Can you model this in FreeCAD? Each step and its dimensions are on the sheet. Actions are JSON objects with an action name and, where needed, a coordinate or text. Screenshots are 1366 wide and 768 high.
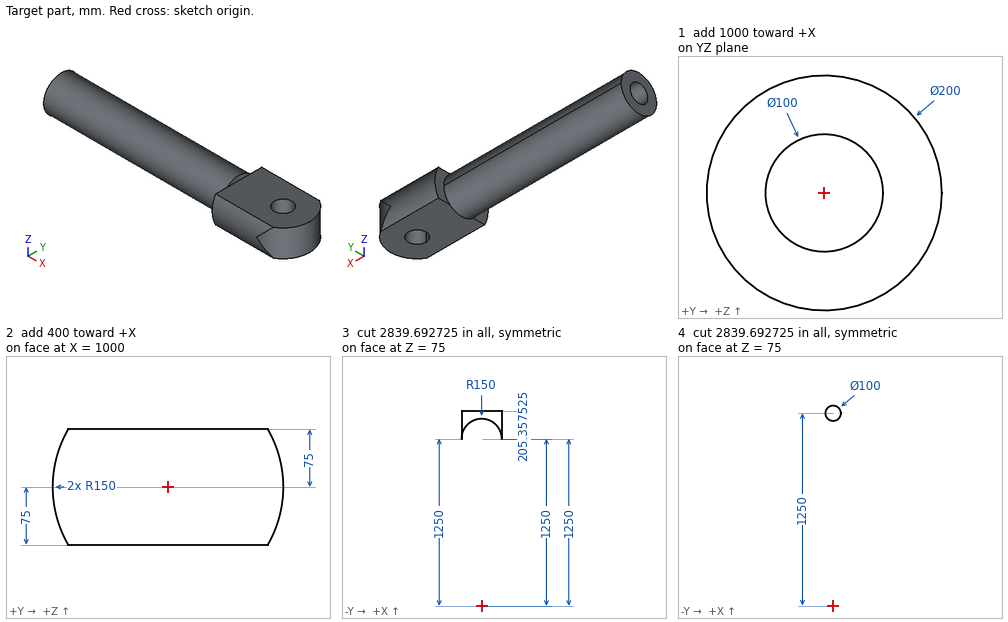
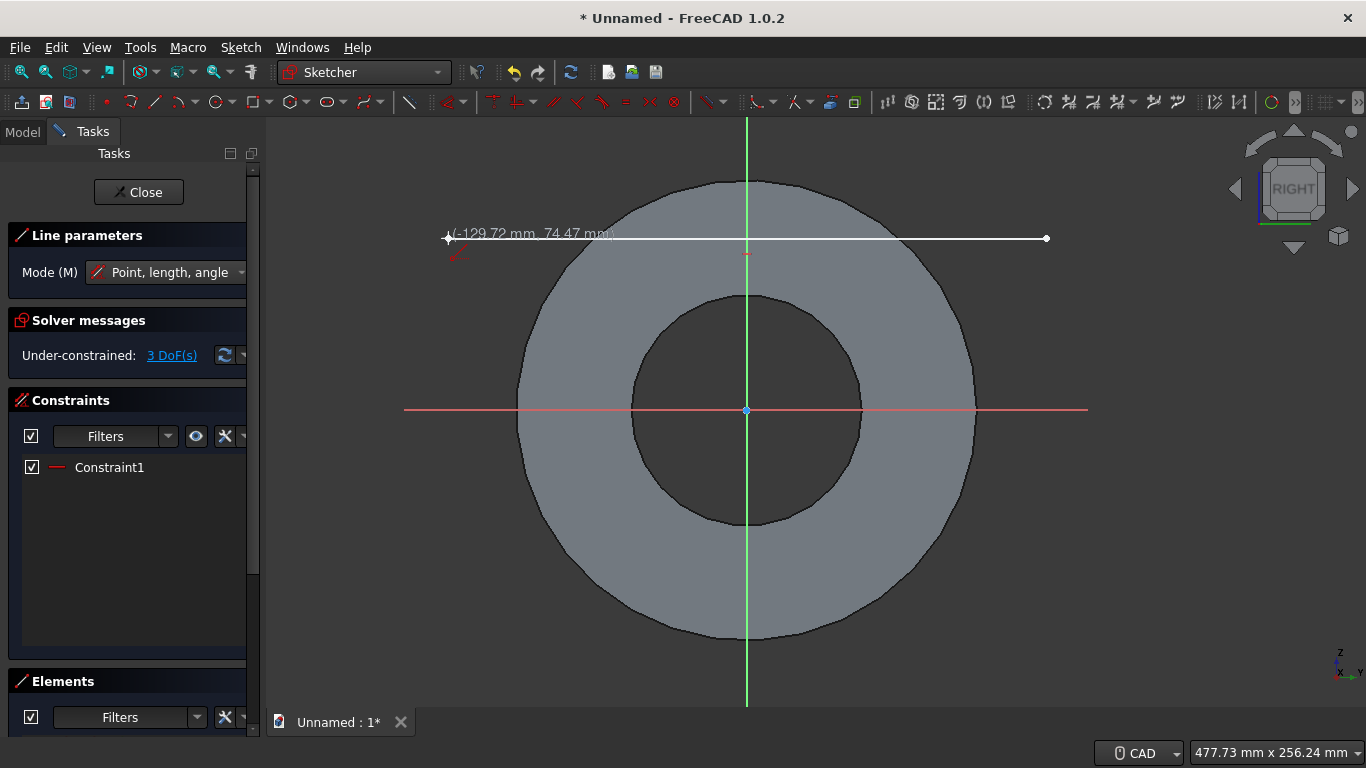
{"action": "left_click", "coordinate": [448, 583]}
{"action": "left_click", "coordinate": [1046, 583]}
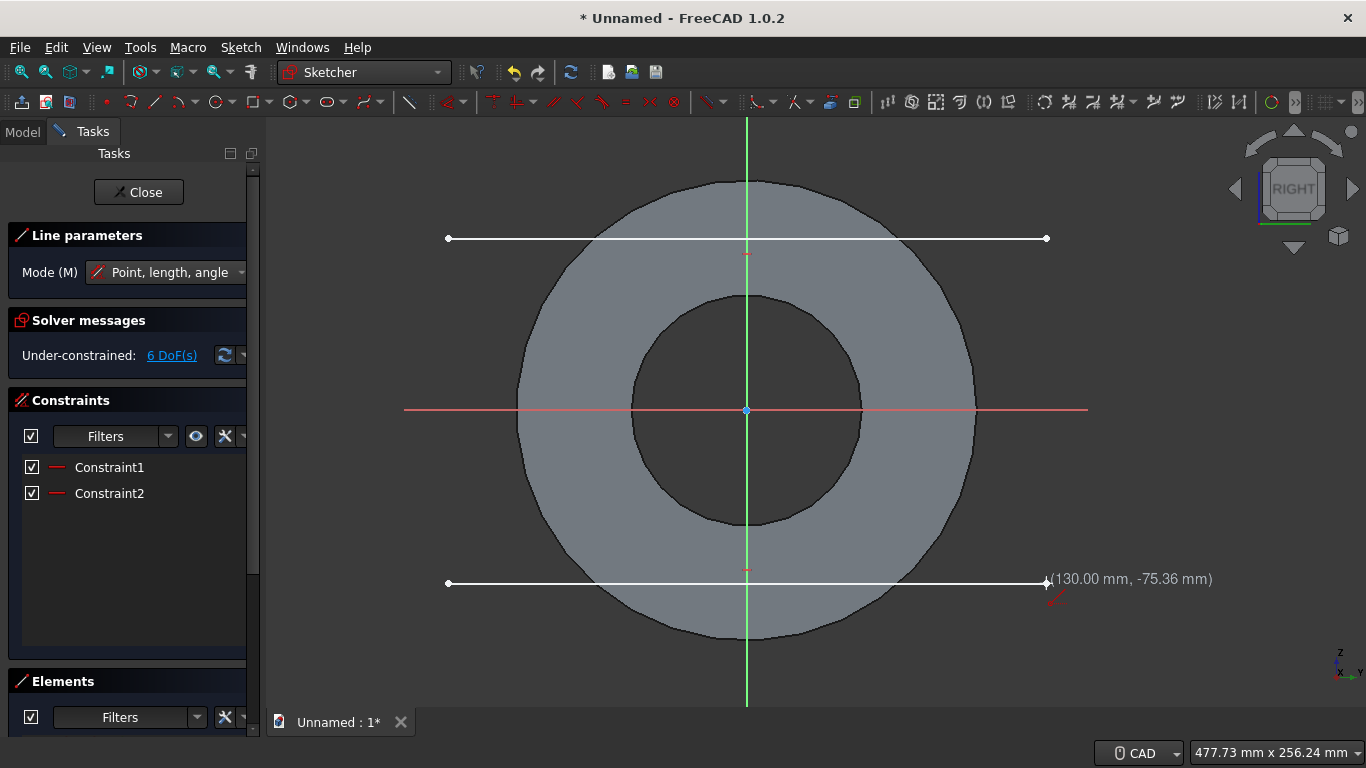
{"action": "key", "text": "g 3 a"}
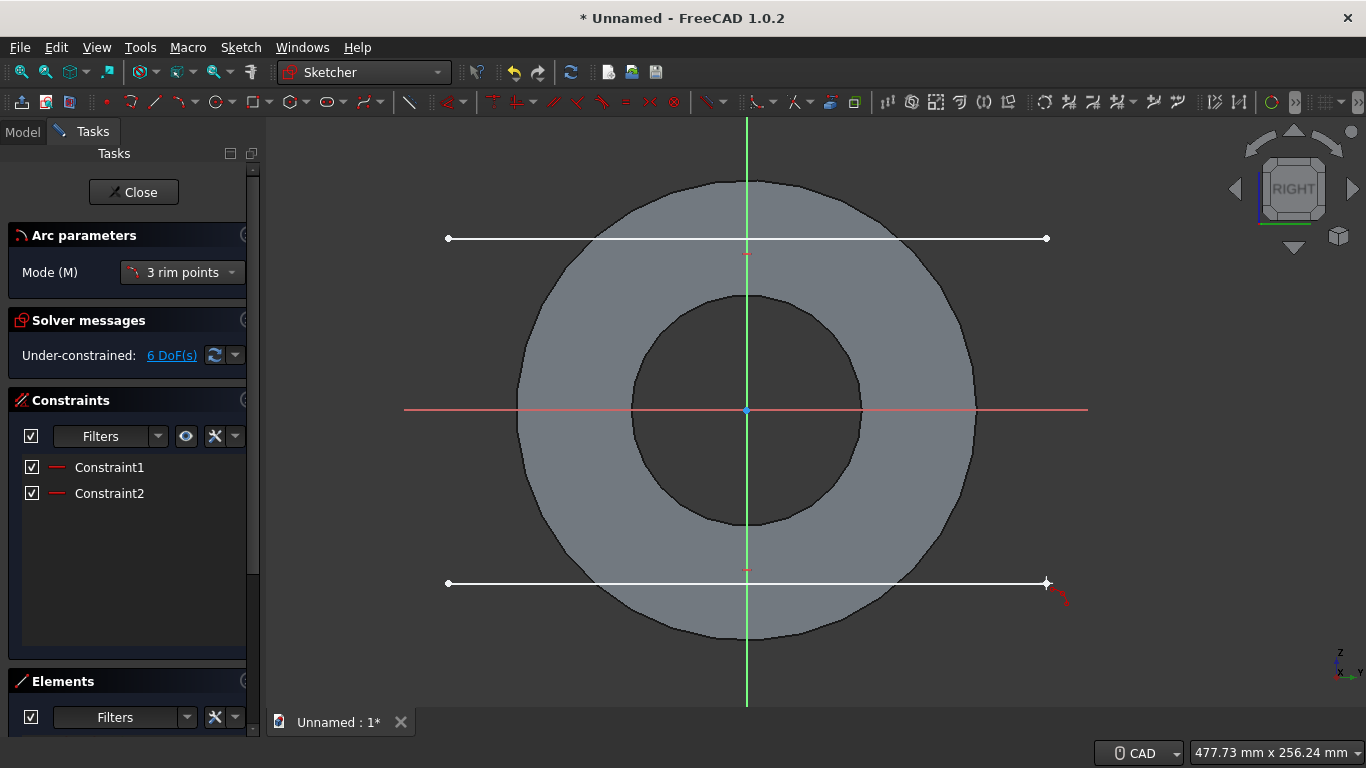
{"action": "left_click", "coordinate": [448, 239]}
{"action": "left_click", "coordinate": [448, 584]}
{"action": "left_click", "coordinate": [403, 374]}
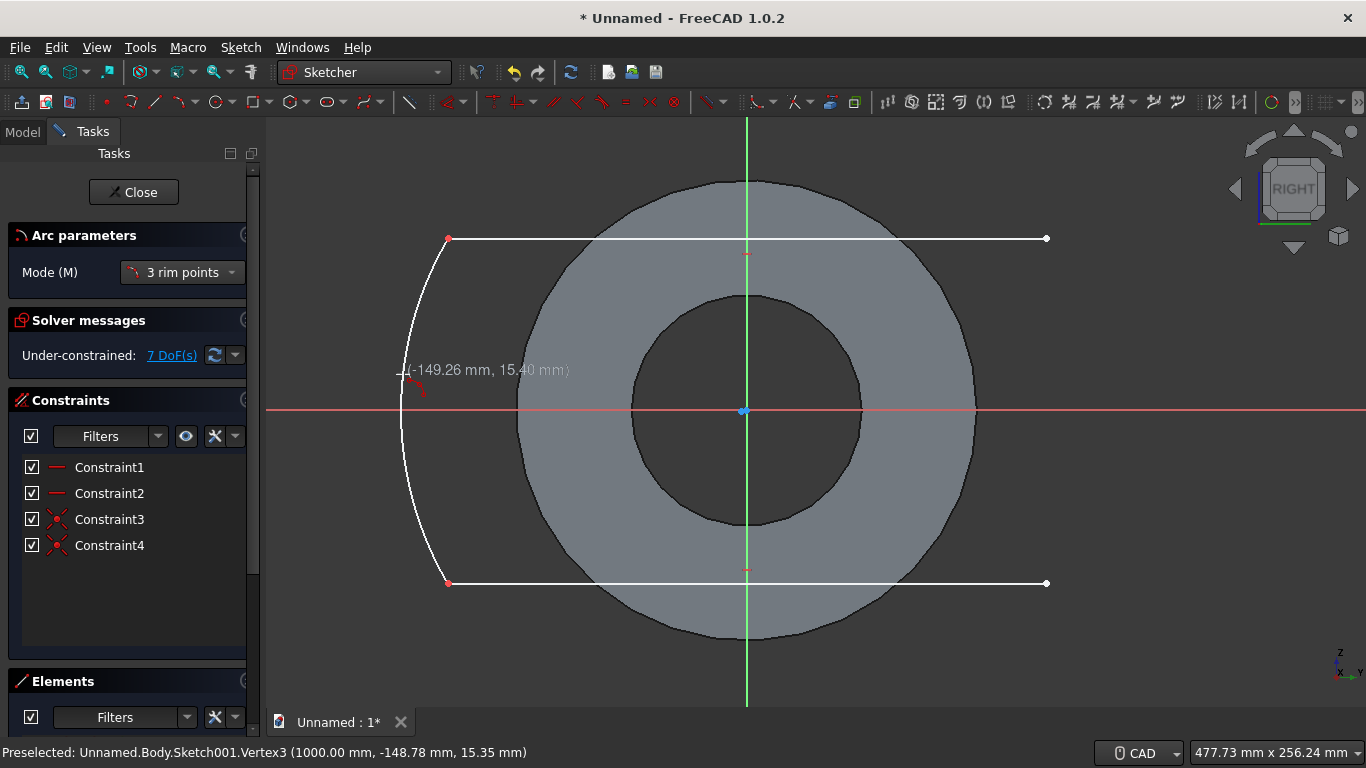
{"action": "left_click", "coordinate": [1046, 584]}
{"action": "left_click", "coordinate": [1046, 239]}
{"action": "left_click", "coordinate": [1090, 447]}
{"action": "key", "text": "Escape"}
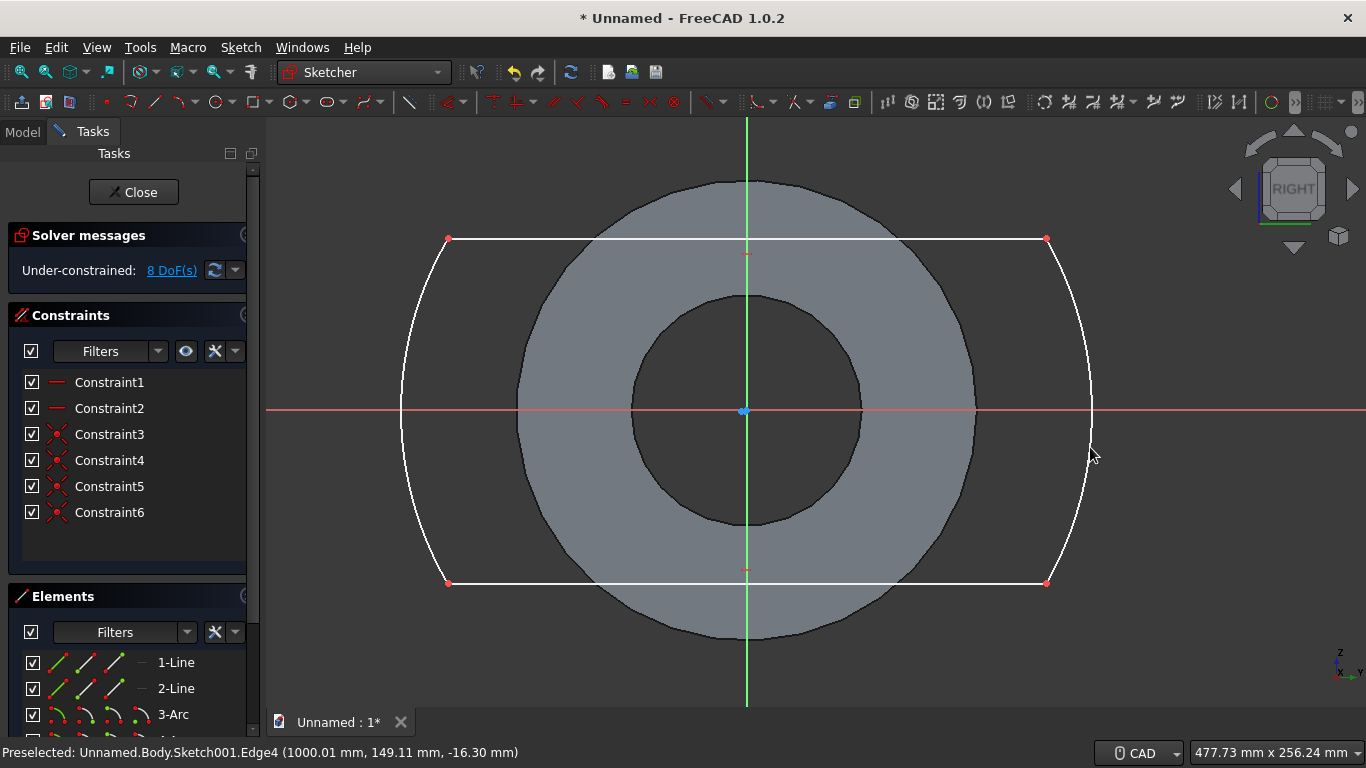
{"action": "left_click", "coordinate": [409, 340]}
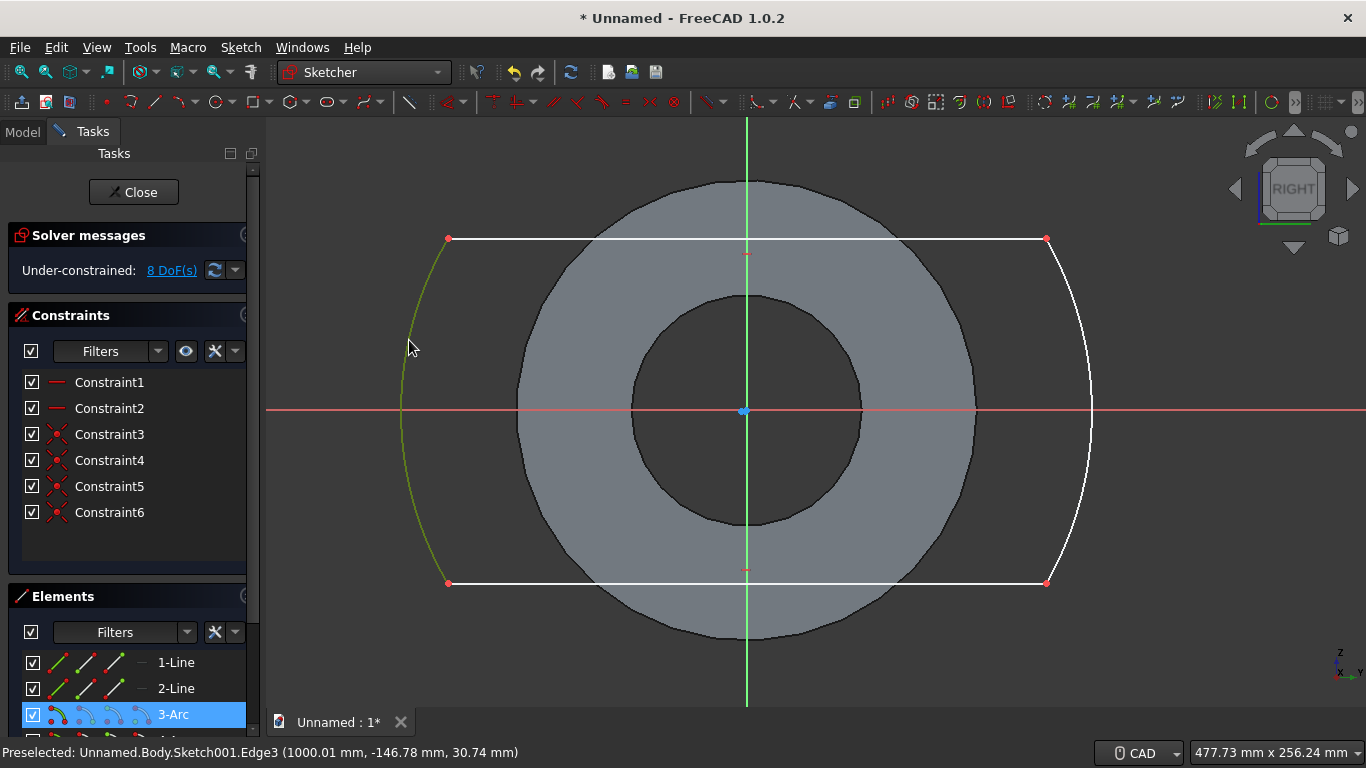
{"action": "left_click", "coordinate": [1084, 483]}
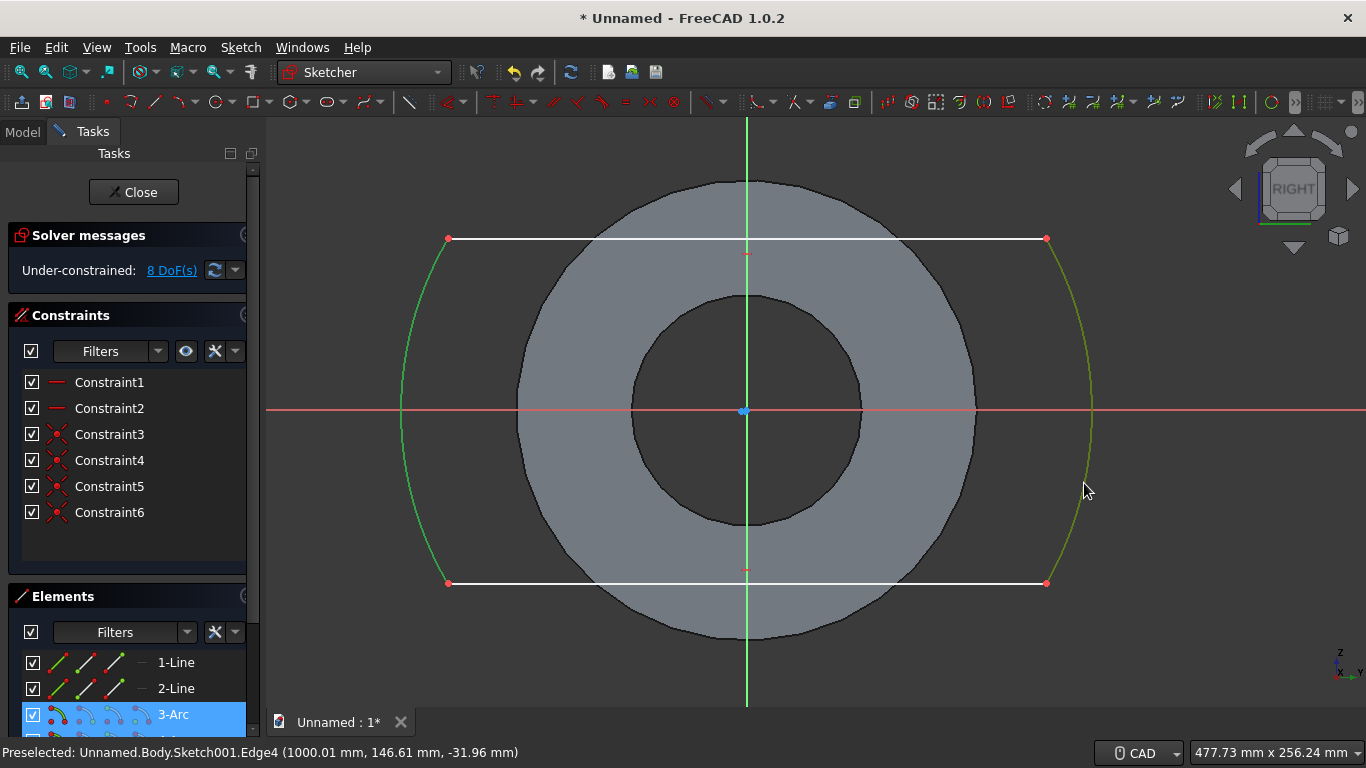
{"action": "left_click", "coordinate": [494, 102]}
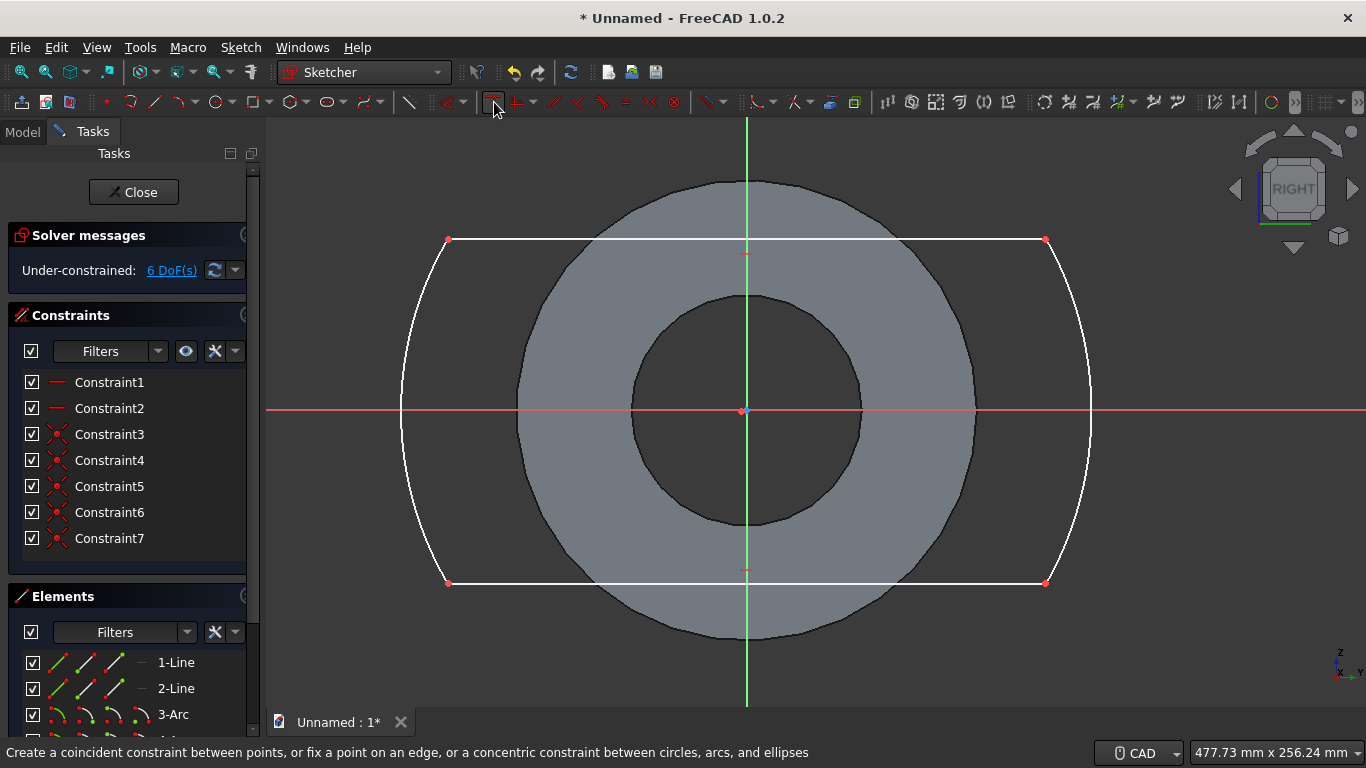
{"action": "left_click_drag", "start_coordinate": [731, 400], "coordinate": [757, 422]}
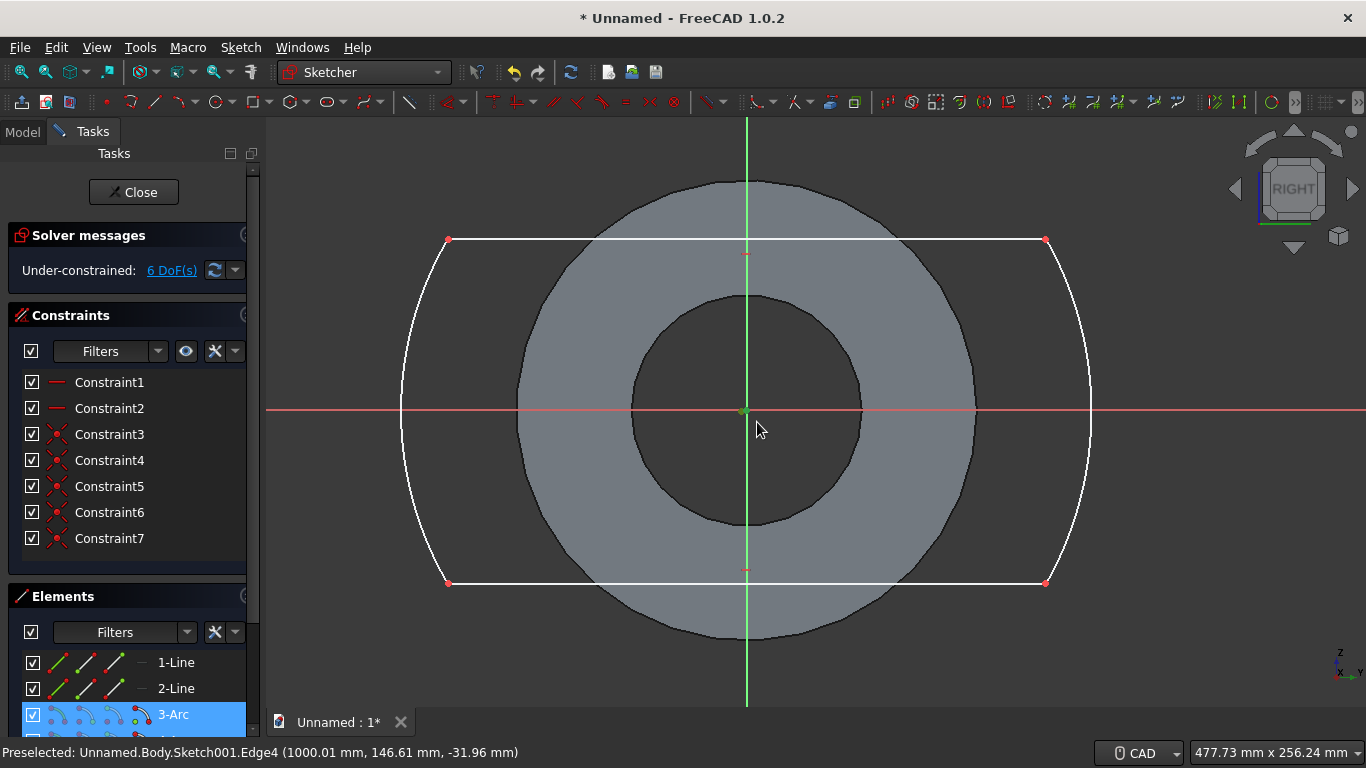
{"action": "left_click", "coordinate": [494, 102]}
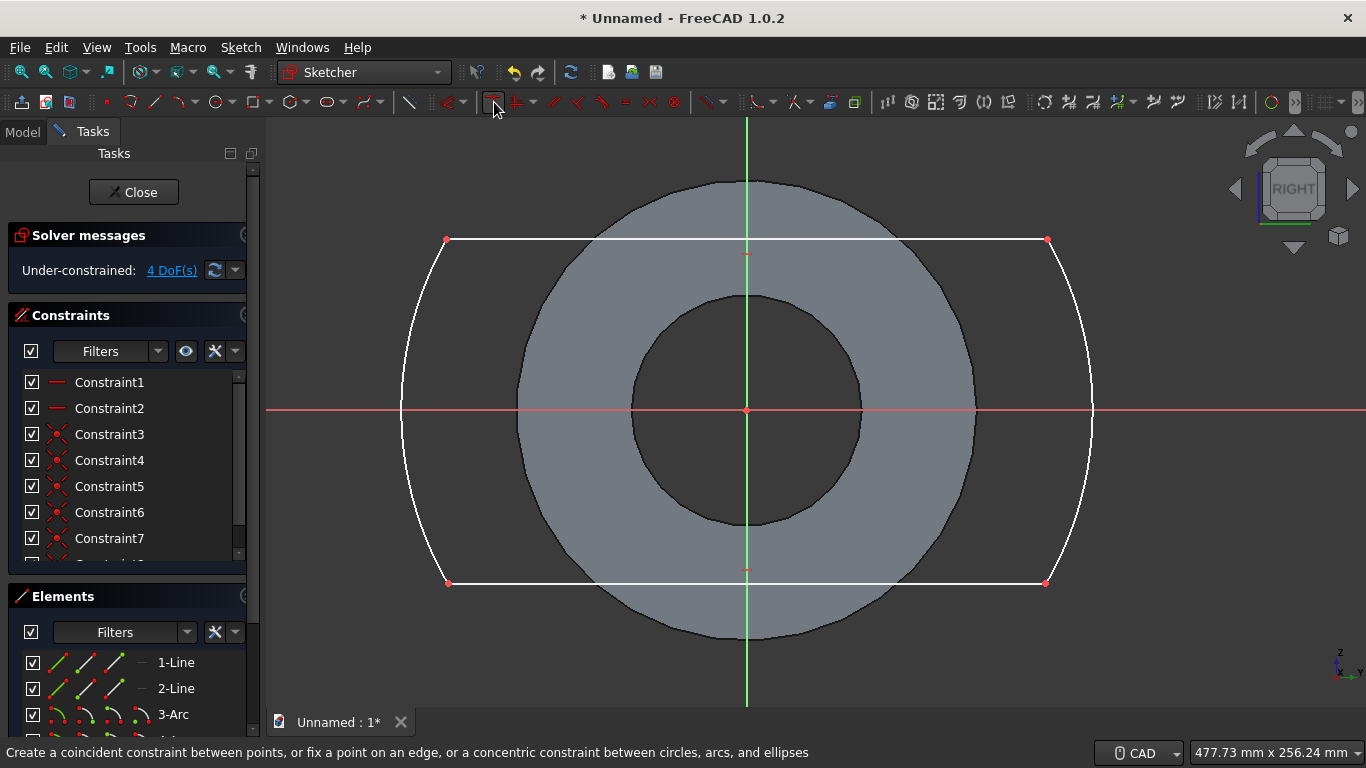
{"action": "left_click", "coordinate": [409, 340]}